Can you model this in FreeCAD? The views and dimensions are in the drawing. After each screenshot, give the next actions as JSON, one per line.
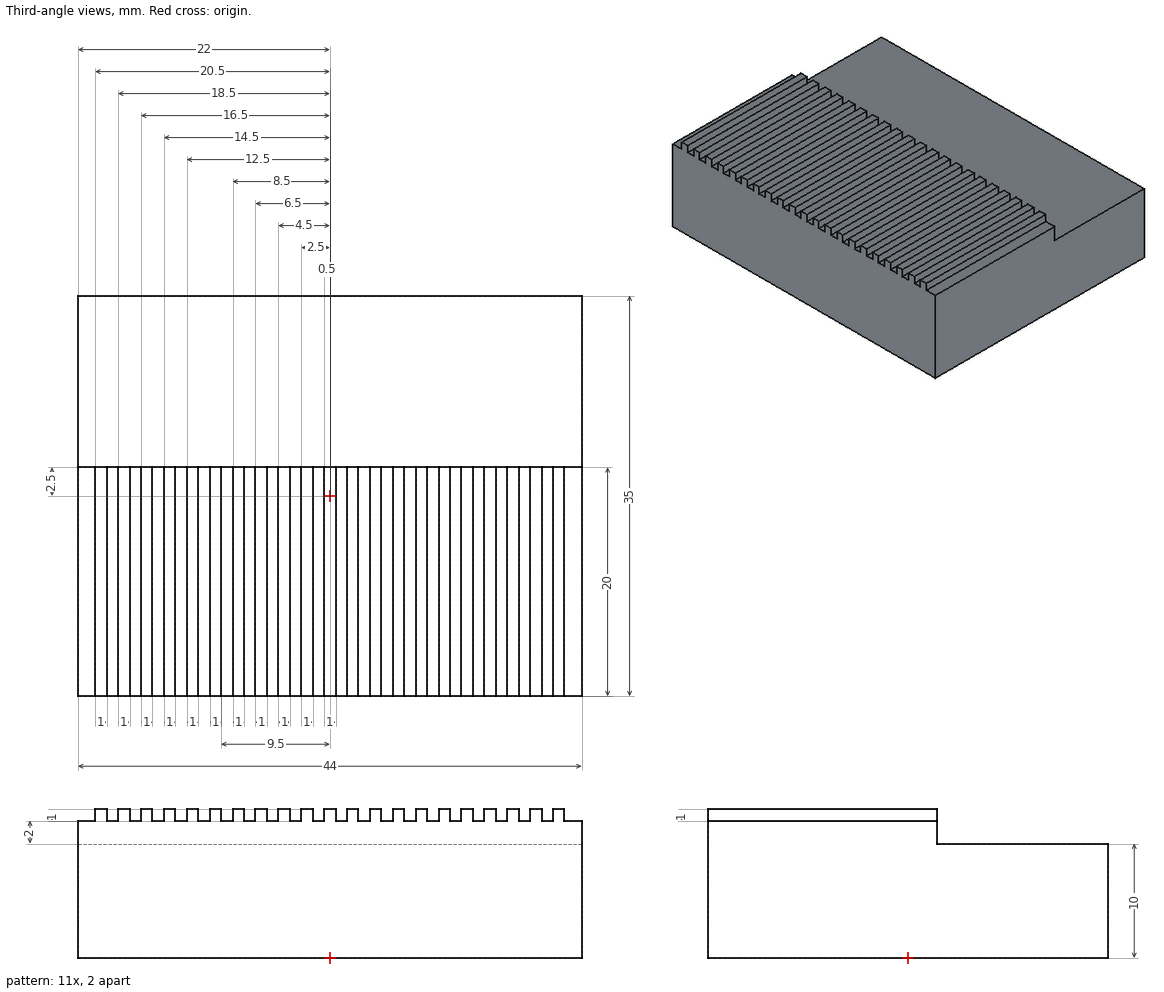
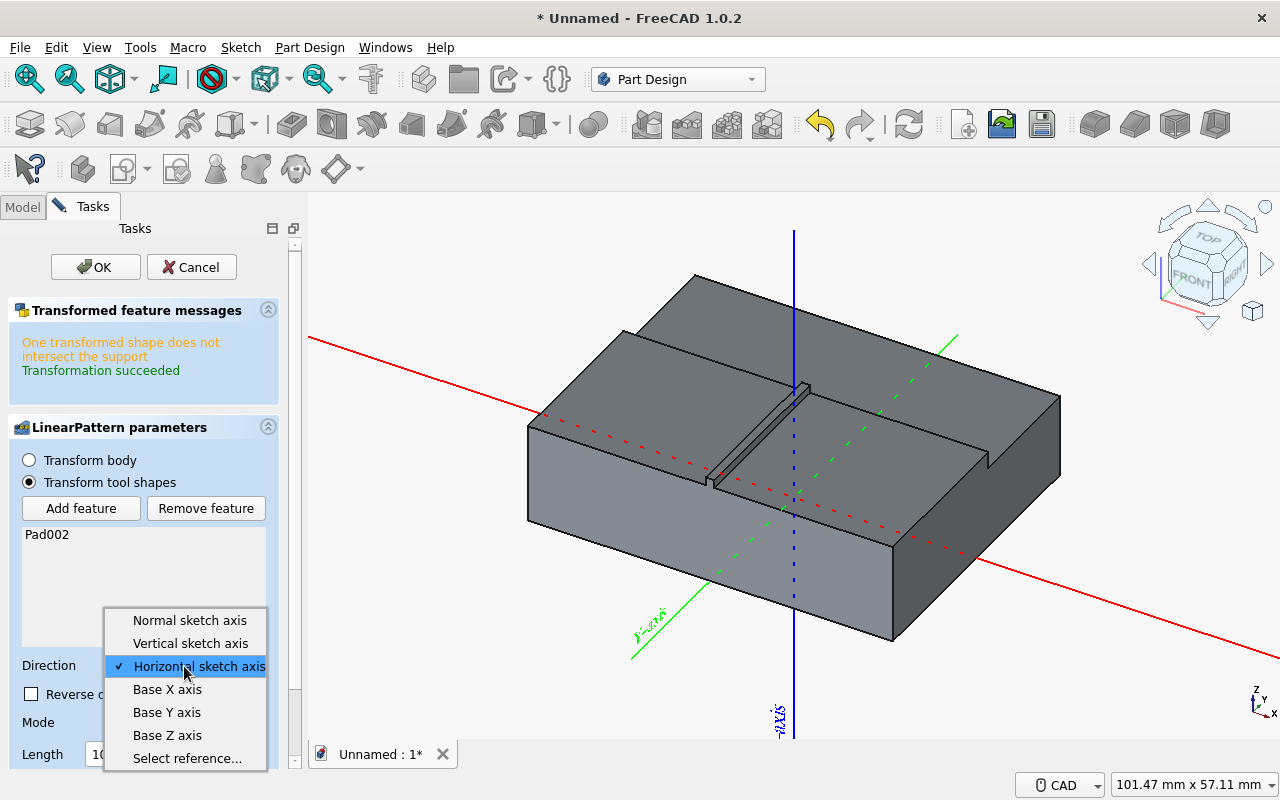
{"action": "left_click", "coordinate": [184, 690]}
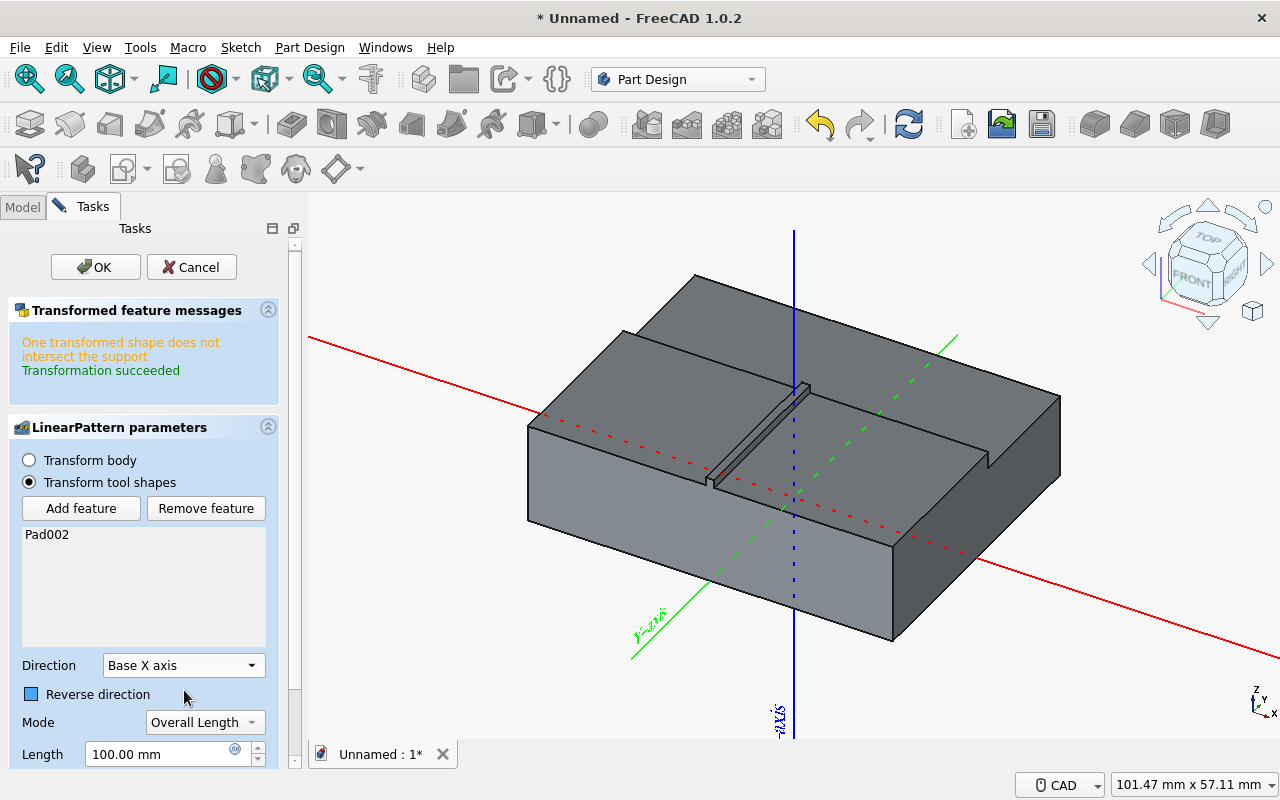
{"action": "left_click", "coordinate": [206, 722]}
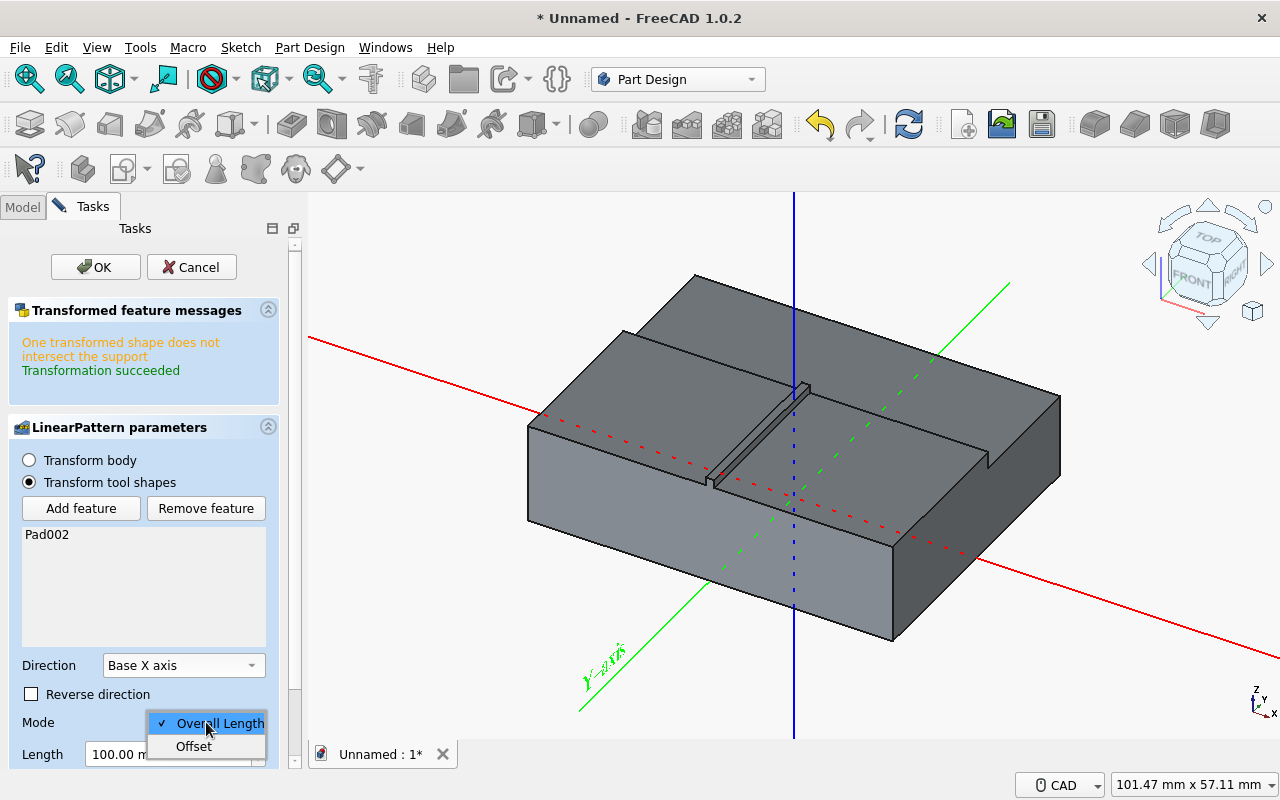
{"action": "left_click", "coordinate": [206, 746]}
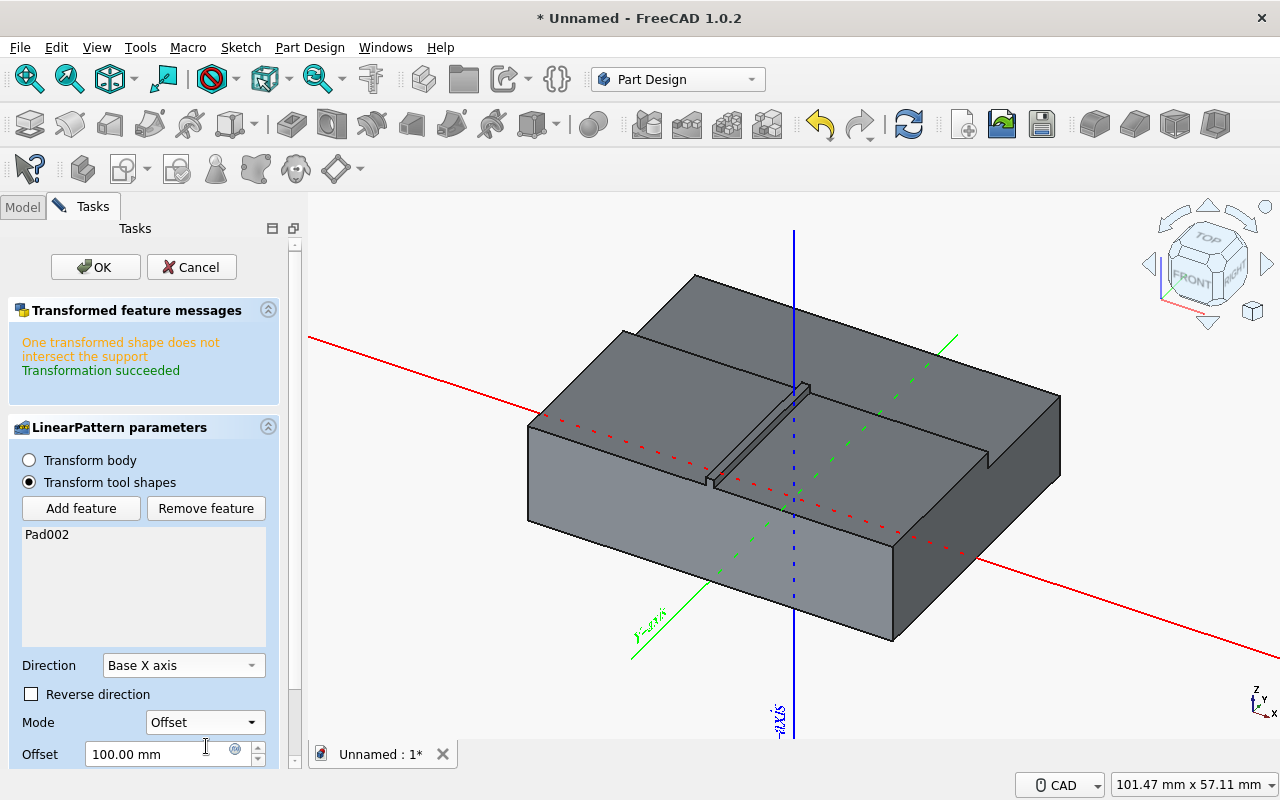
{"action": "triple_click", "coordinate": [168, 754]}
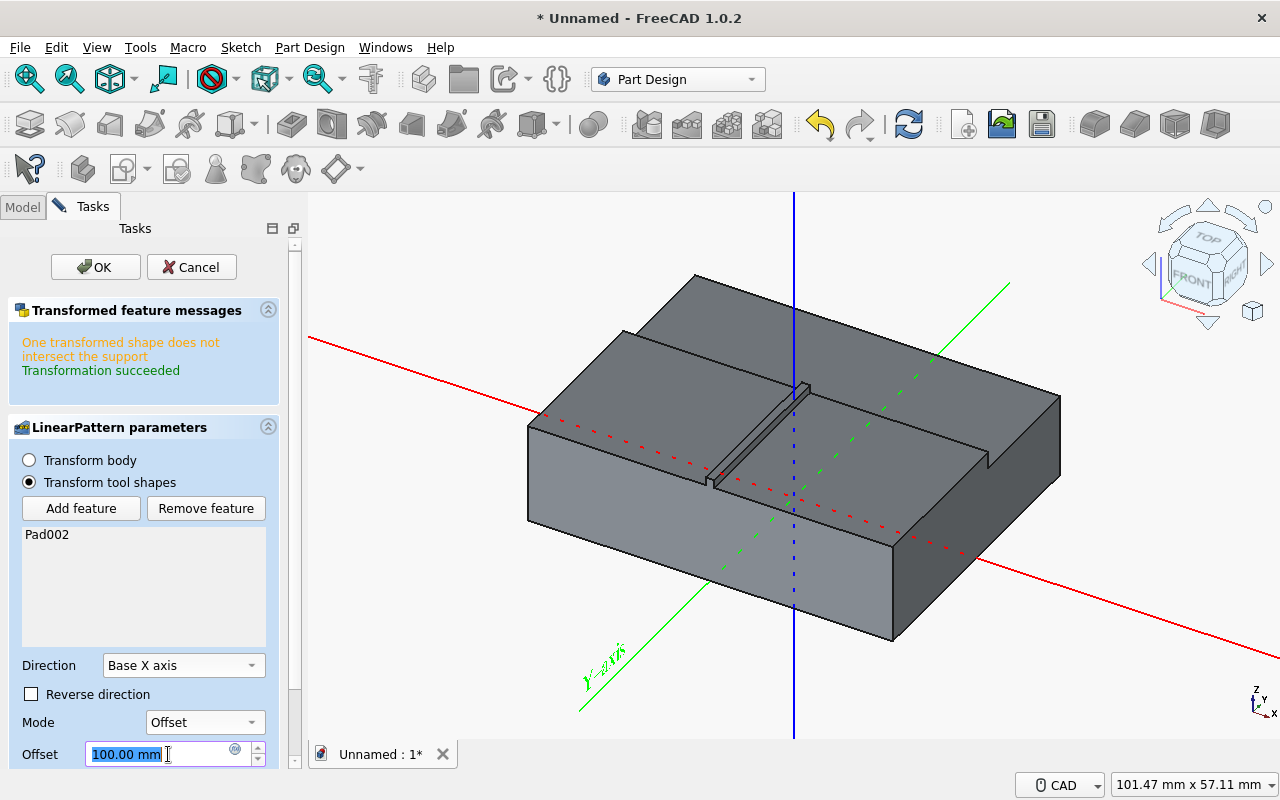
{"action": "type", "text": "2"}
{"action": "key", "text": "Tab"}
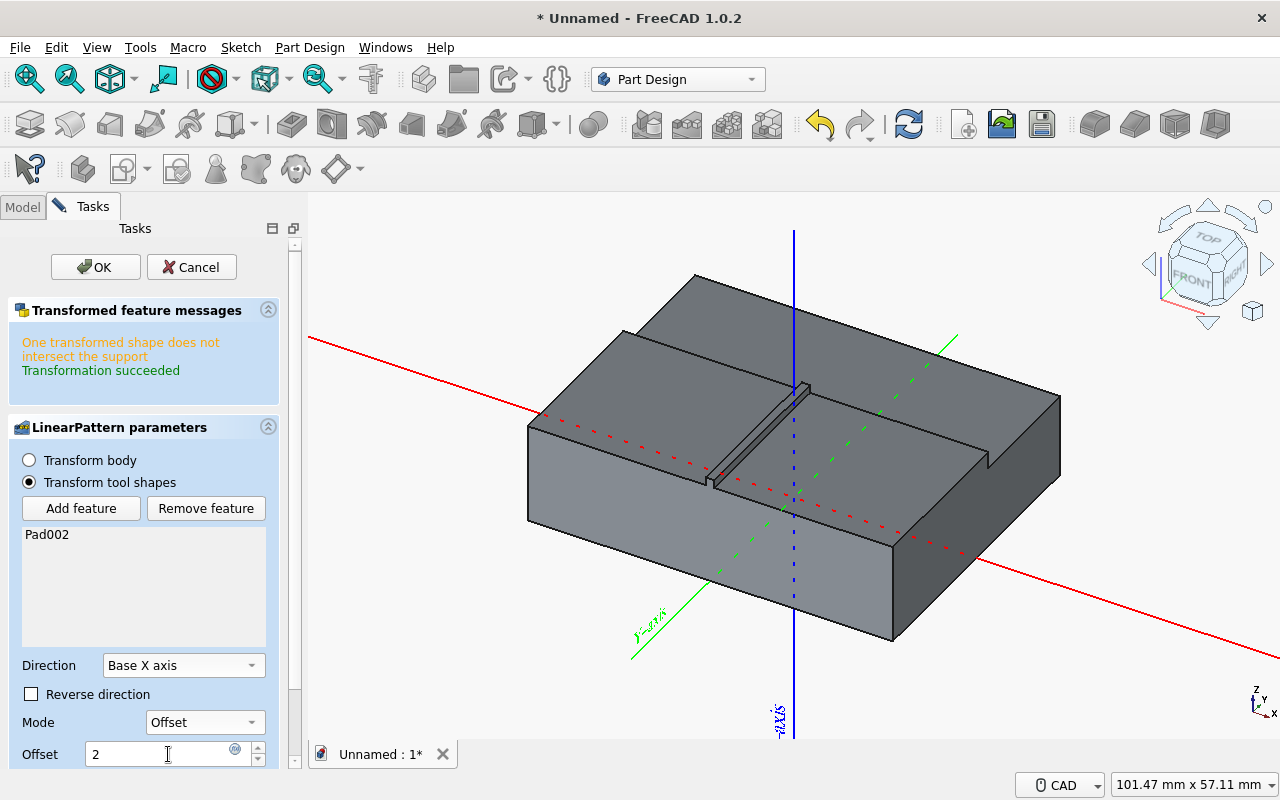
{"action": "scroll", "coordinate": [295, 503], "scroll_direction": "down", "scroll_amount": 2}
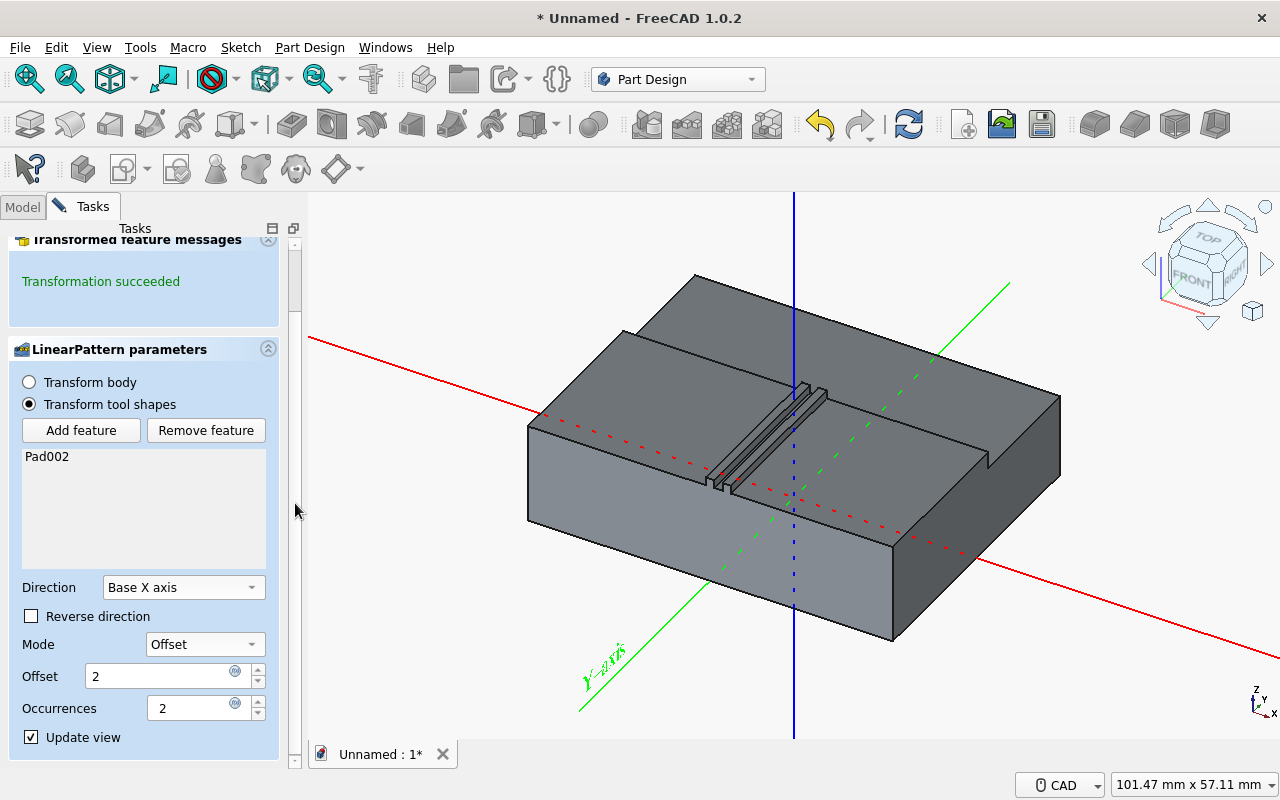
{"action": "triple_click", "coordinate": [198, 708]}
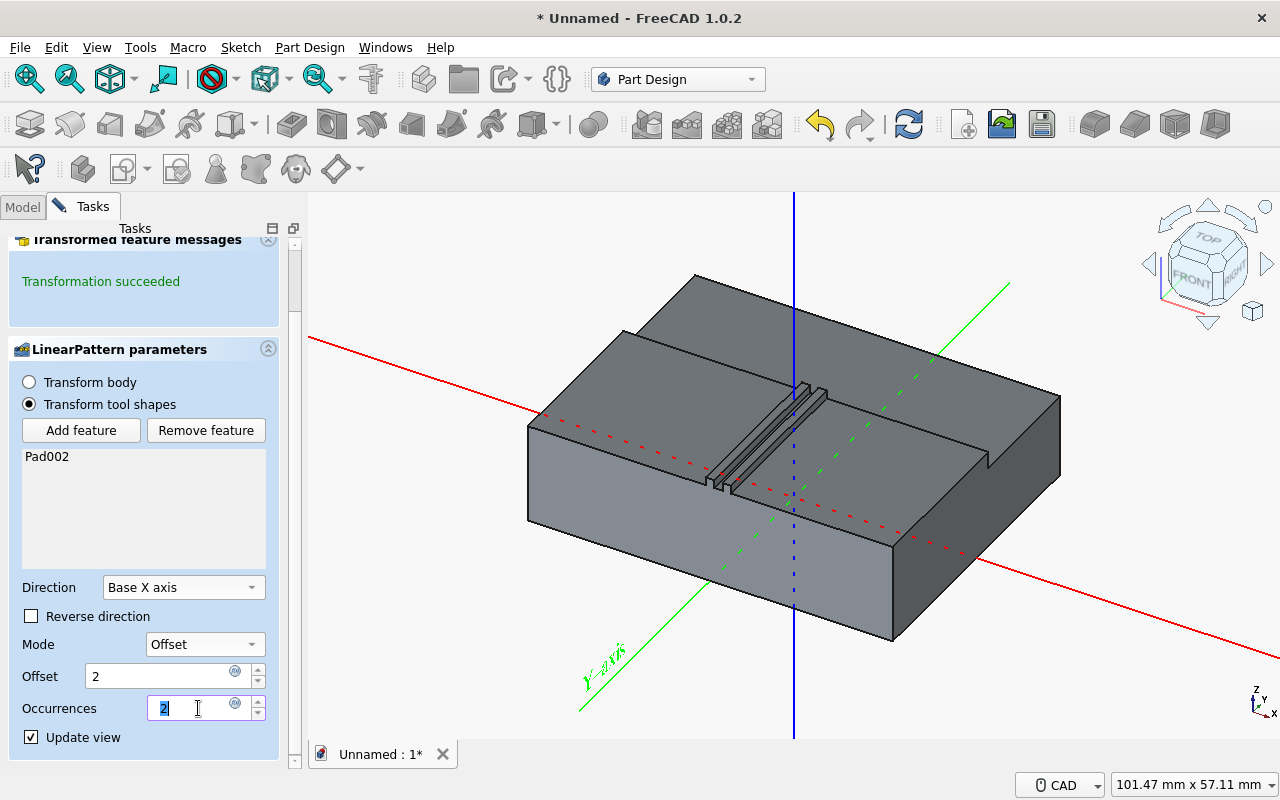
{"action": "type", "text": "11"}
{"action": "key", "text": "Tab"}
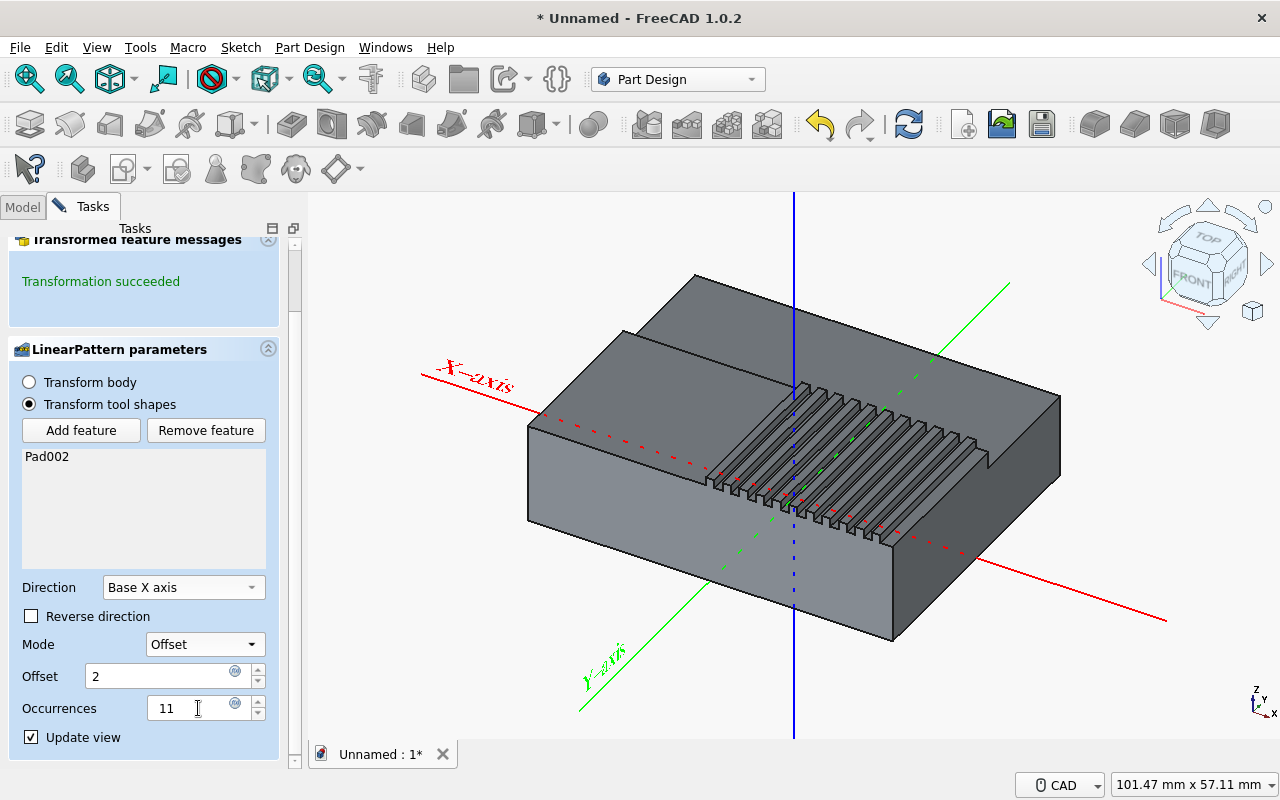
{"action": "scroll", "coordinate": [295, 503], "scroll_direction": "up", "scroll_amount": 2}